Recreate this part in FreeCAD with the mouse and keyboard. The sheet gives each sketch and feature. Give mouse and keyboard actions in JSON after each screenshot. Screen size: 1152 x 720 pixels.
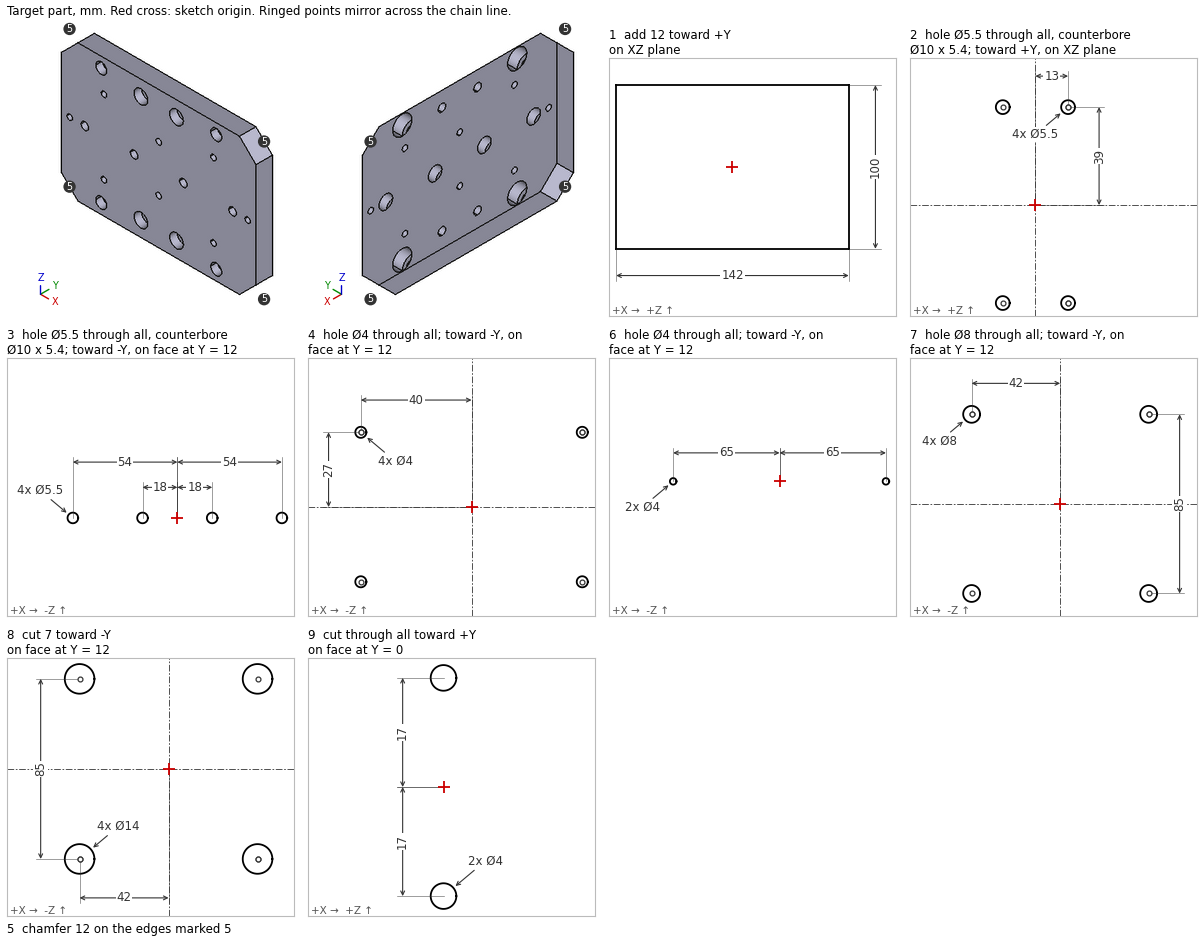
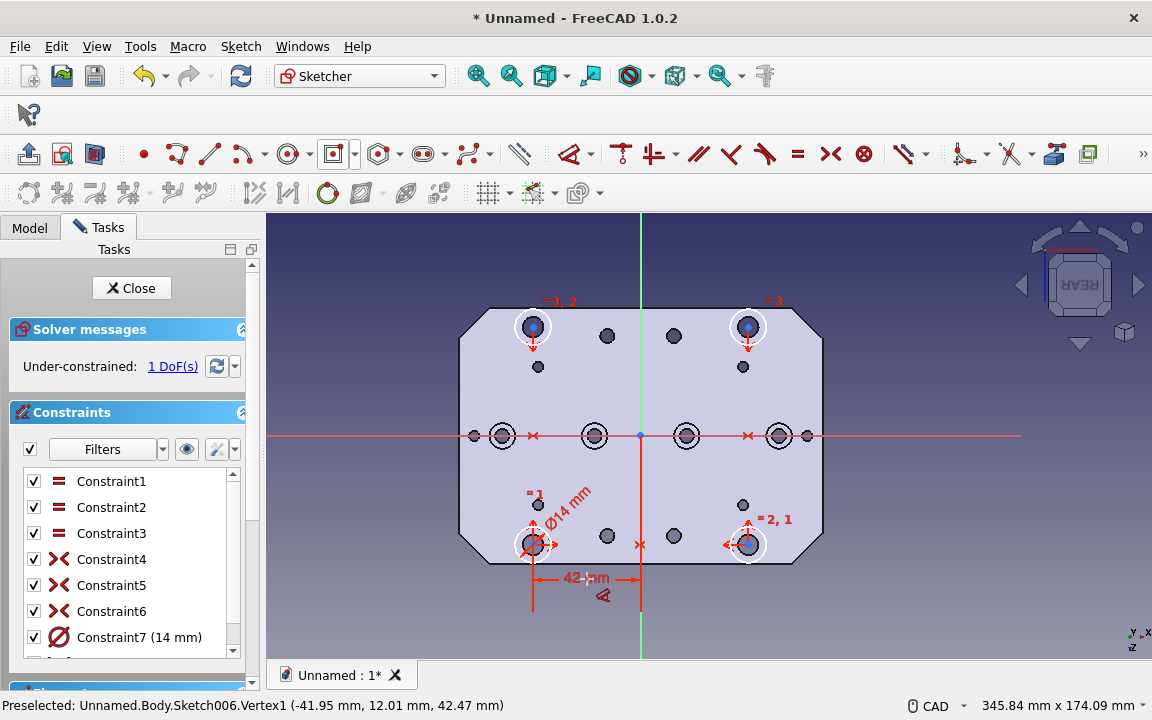
{"action": "left_click", "coordinate": [533, 545]}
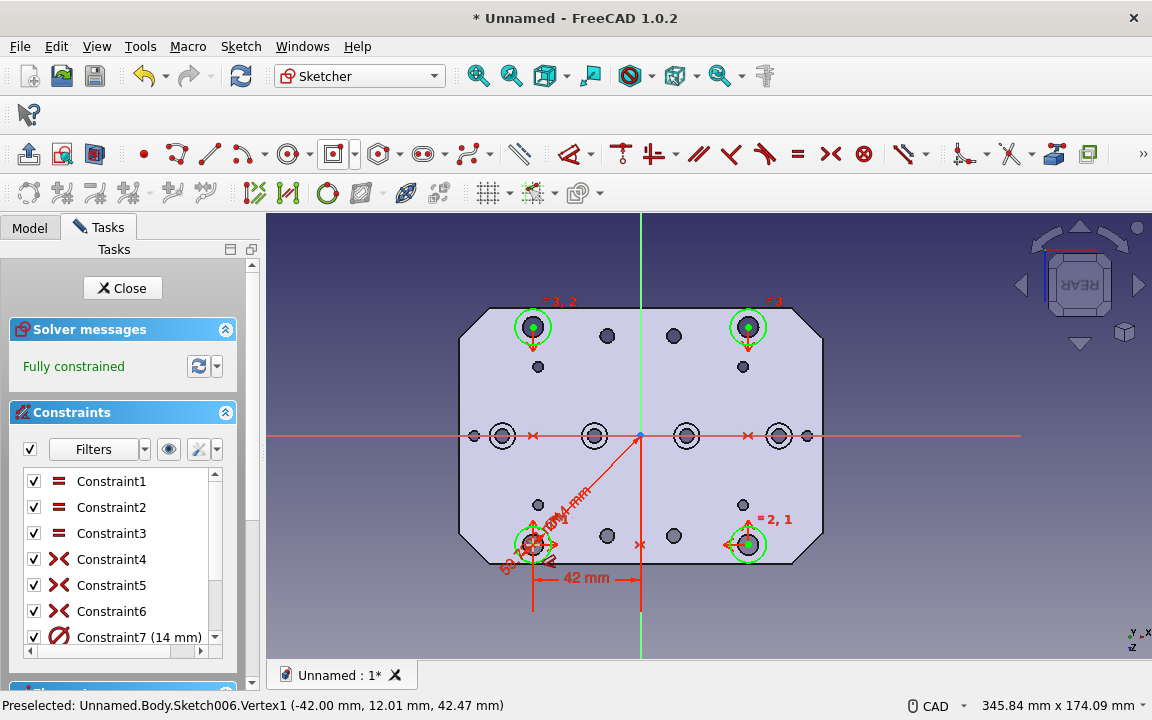
{"action": "left_click", "coordinate": [533, 327]}
{"action": "left_click", "coordinate": [499, 386]}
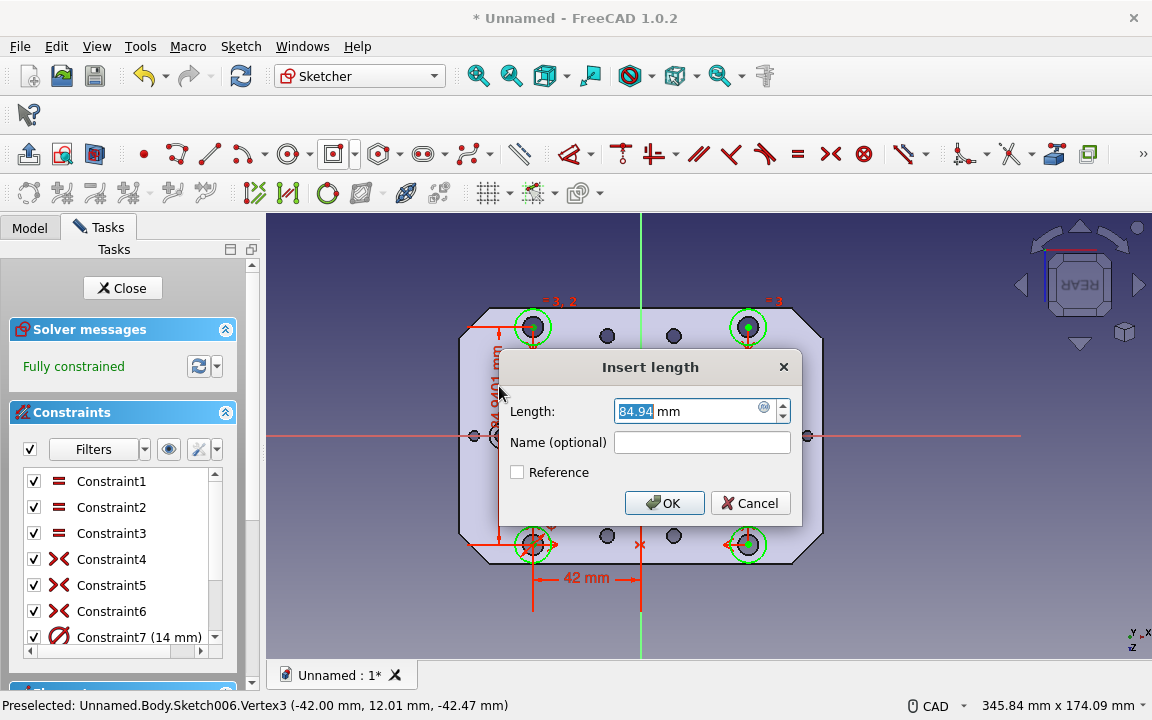
{"action": "type", "text": "85"}
{"action": "key", "text": "Return"}
{"action": "key", "text": "Escape"}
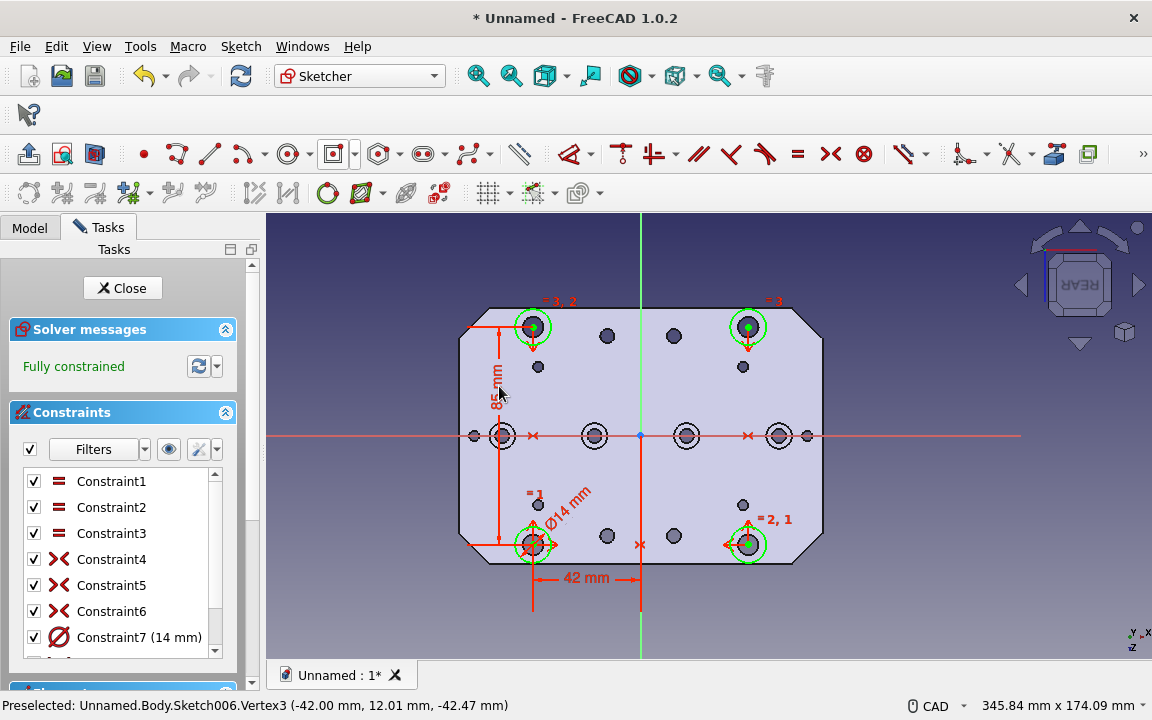
{"action": "left_click", "coordinate": [123, 288]}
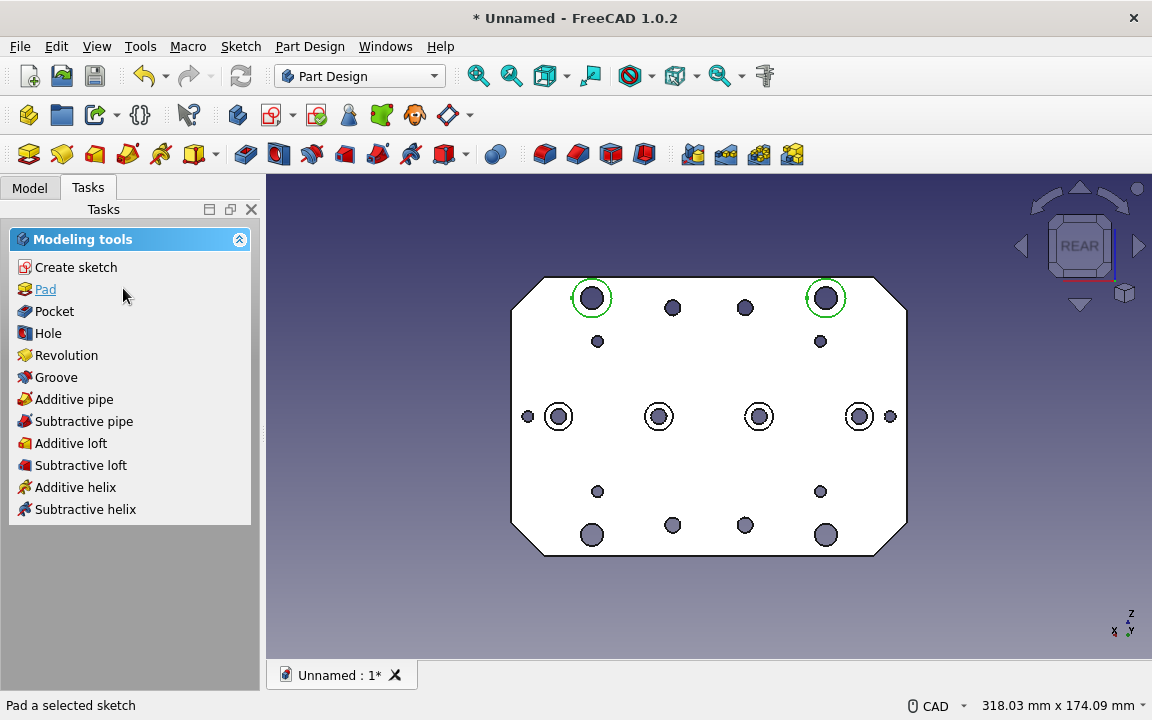
{"action": "left_click", "coordinate": [246, 154]}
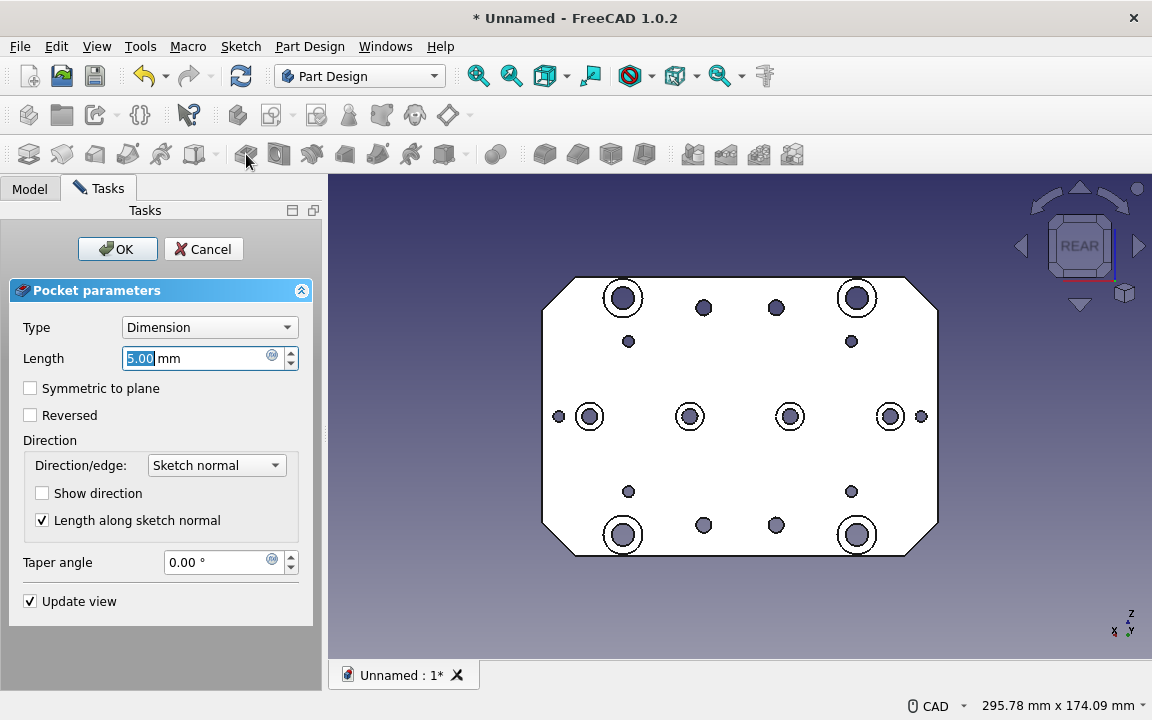
{"action": "type", "text": "7"}
{"action": "key", "text": "Tab"}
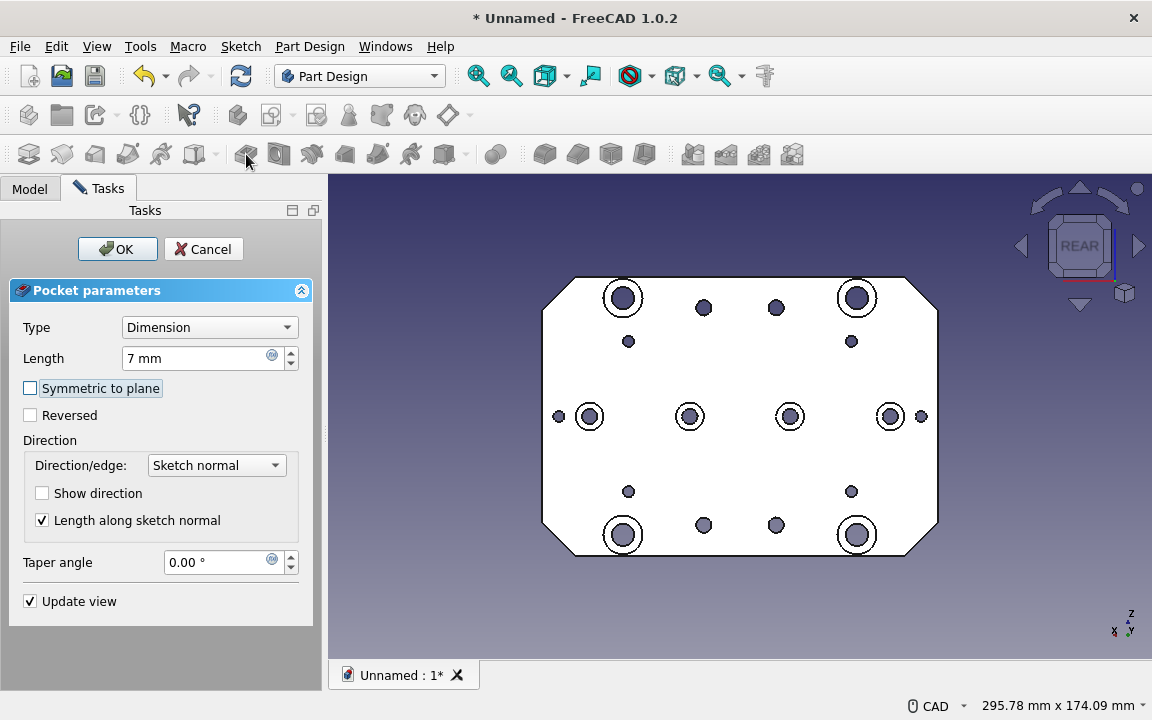
{"action": "left_click", "coordinate": [118, 249]}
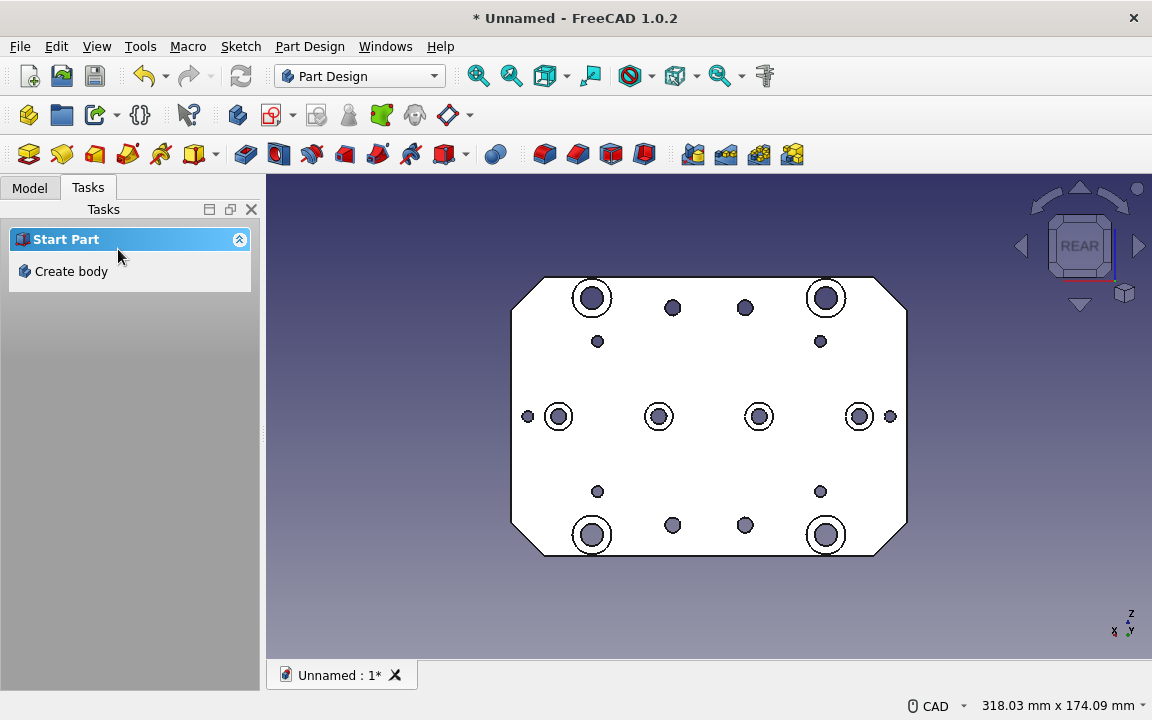
{"action": "key", "text": "0"}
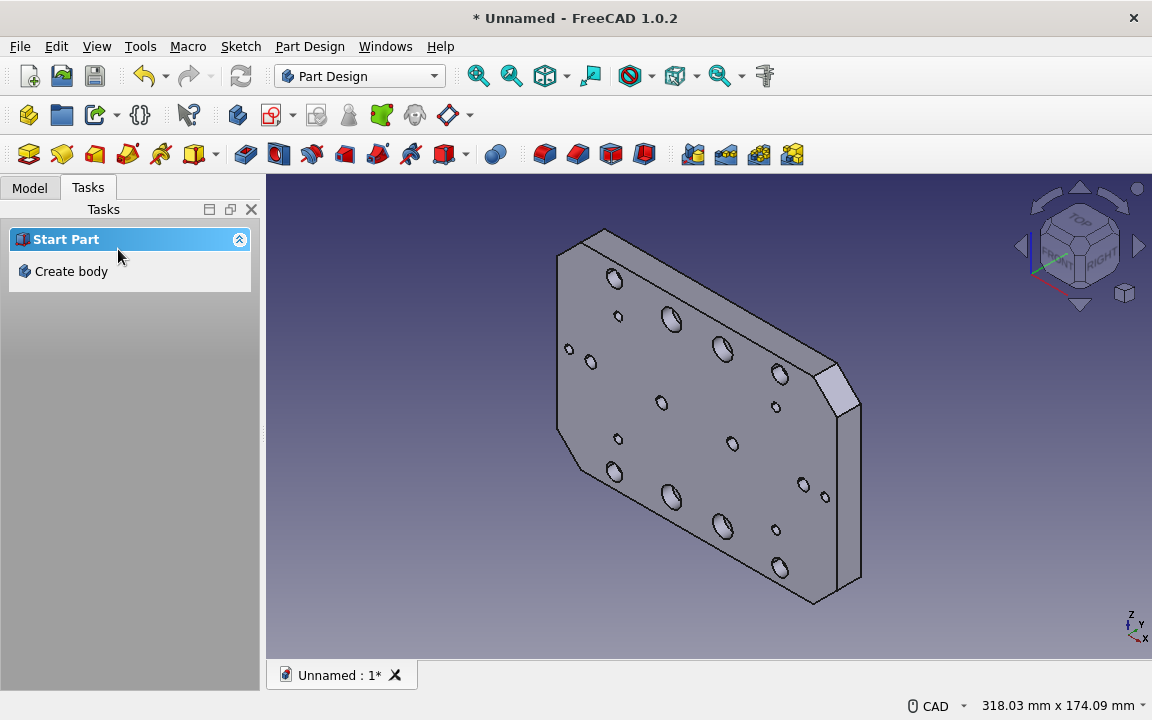
{"action": "left_click", "coordinate": [697, 390]}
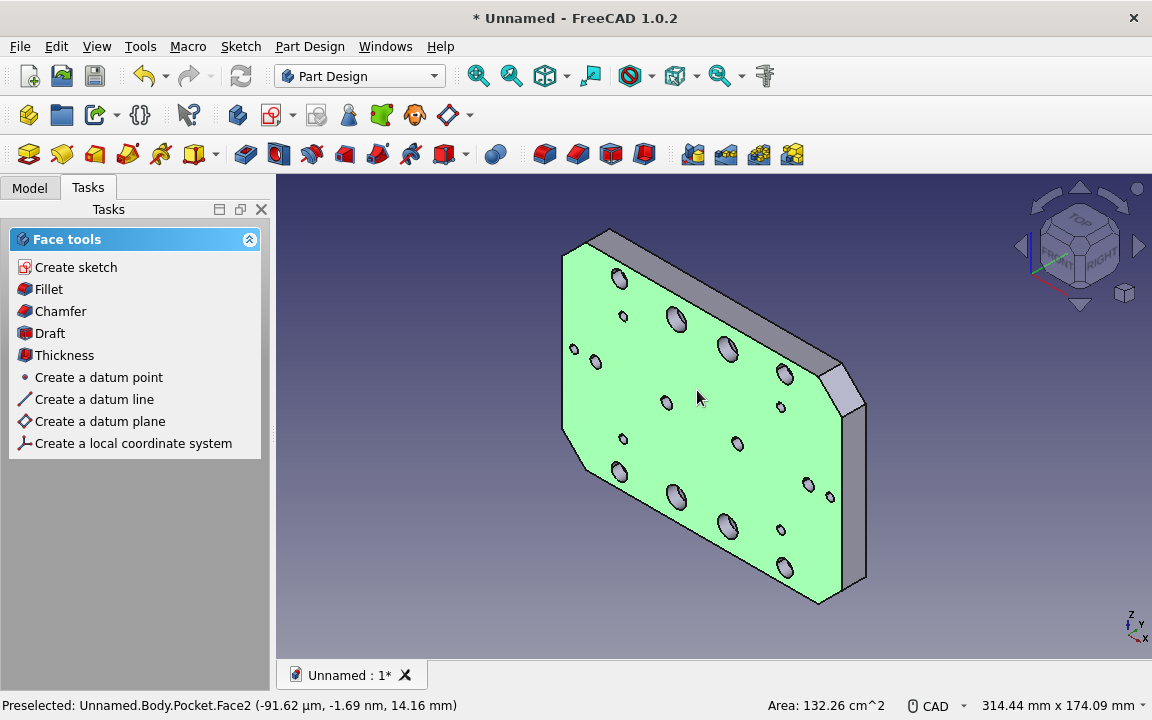
{"action": "left_click", "coordinate": [270, 116]}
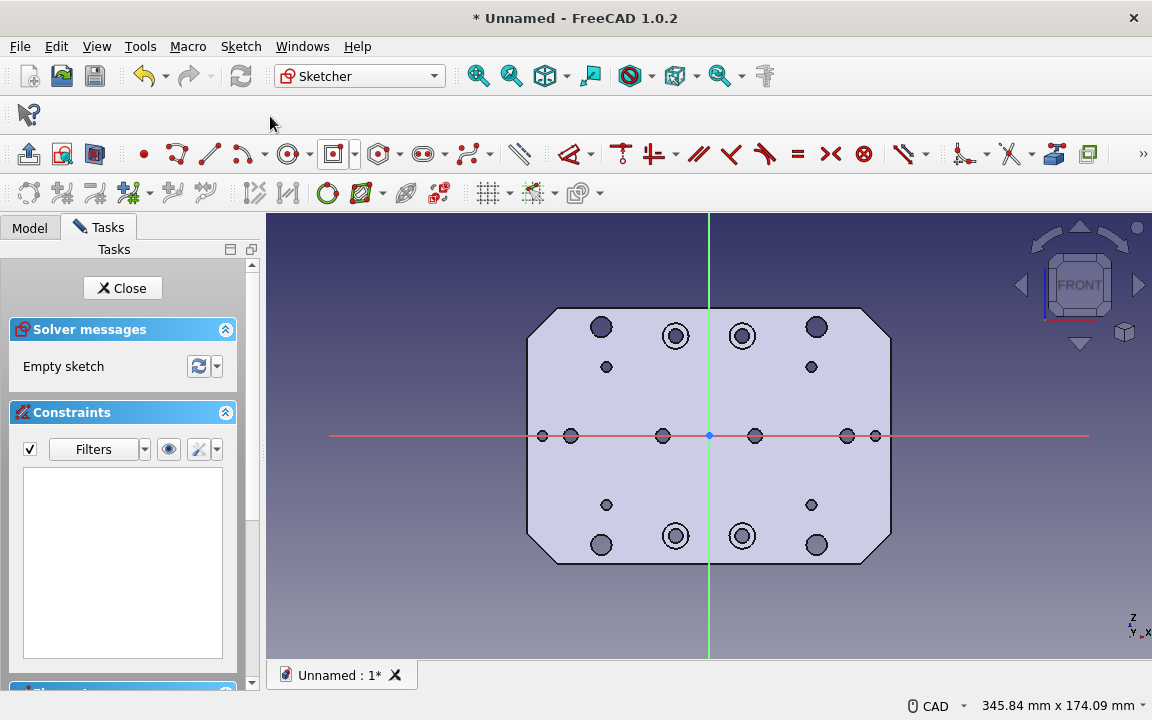
{"action": "scroll", "coordinate": [749, 436], "scroll_direction": "up", "scroll_amount": 5}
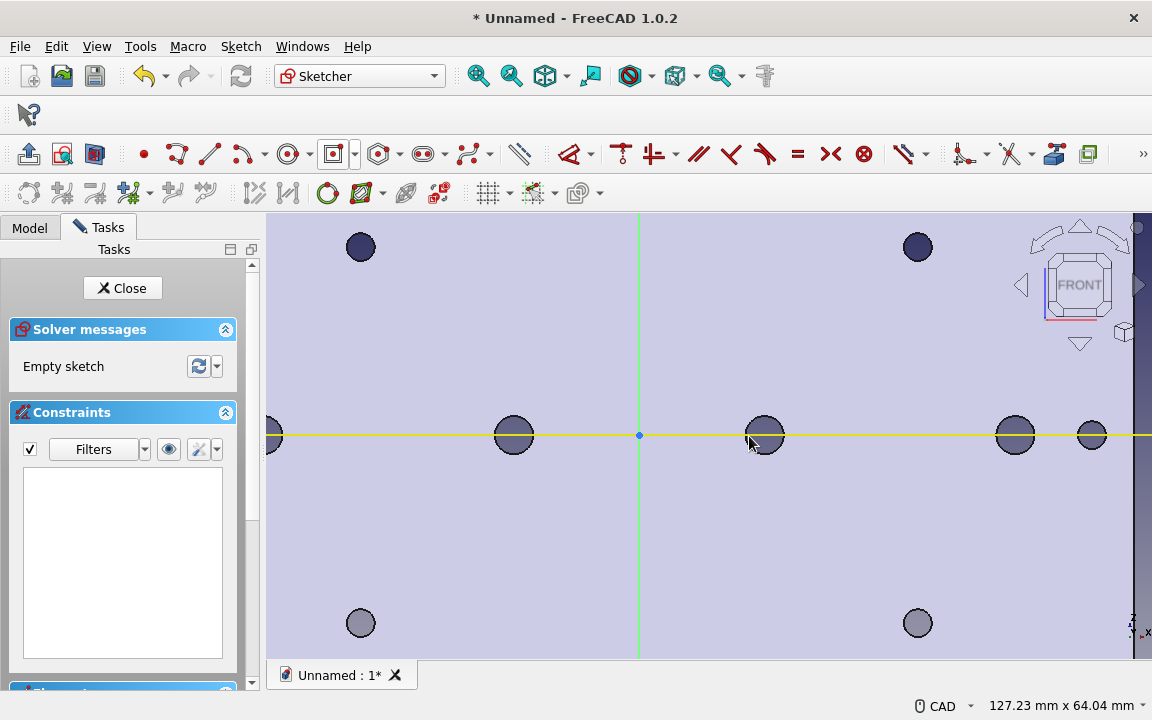
{"action": "left_click", "coordinate": [288, 154]}